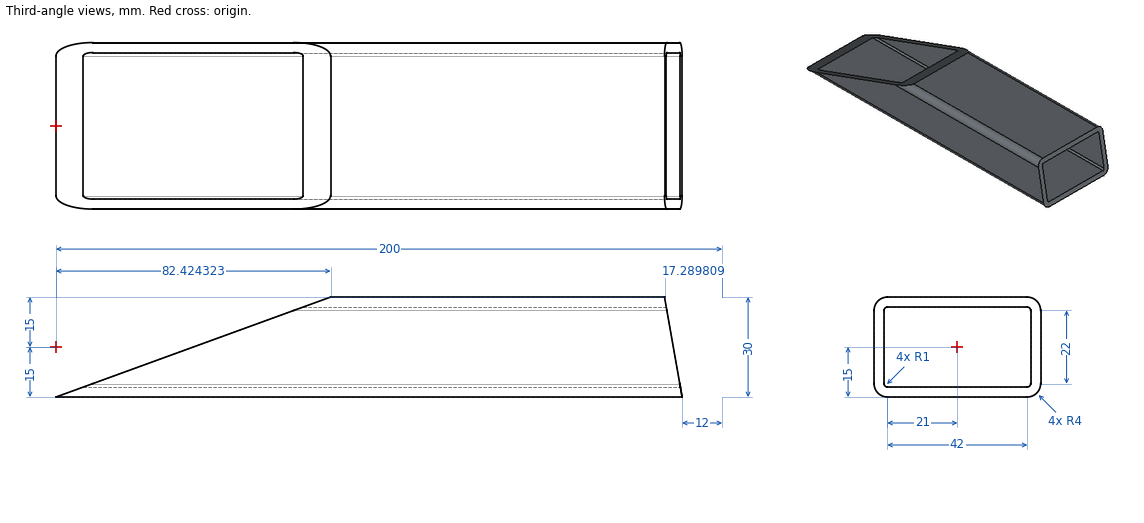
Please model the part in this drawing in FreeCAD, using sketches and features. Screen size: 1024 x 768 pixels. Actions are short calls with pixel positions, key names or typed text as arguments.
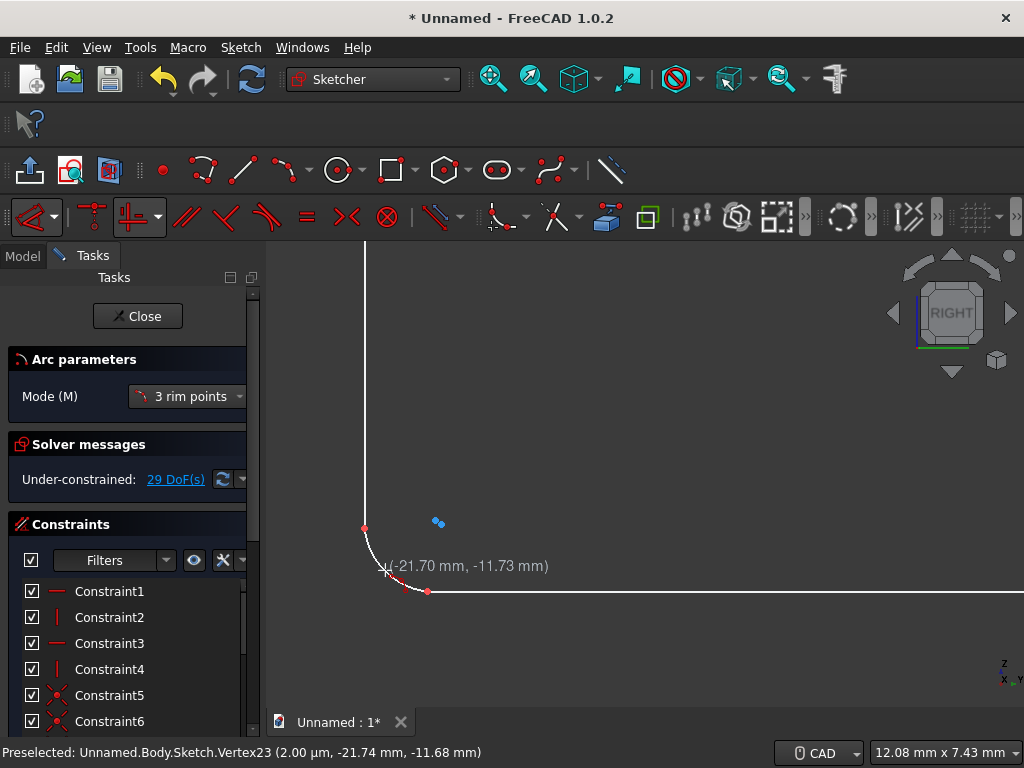
scroll(393, 574, down, 10)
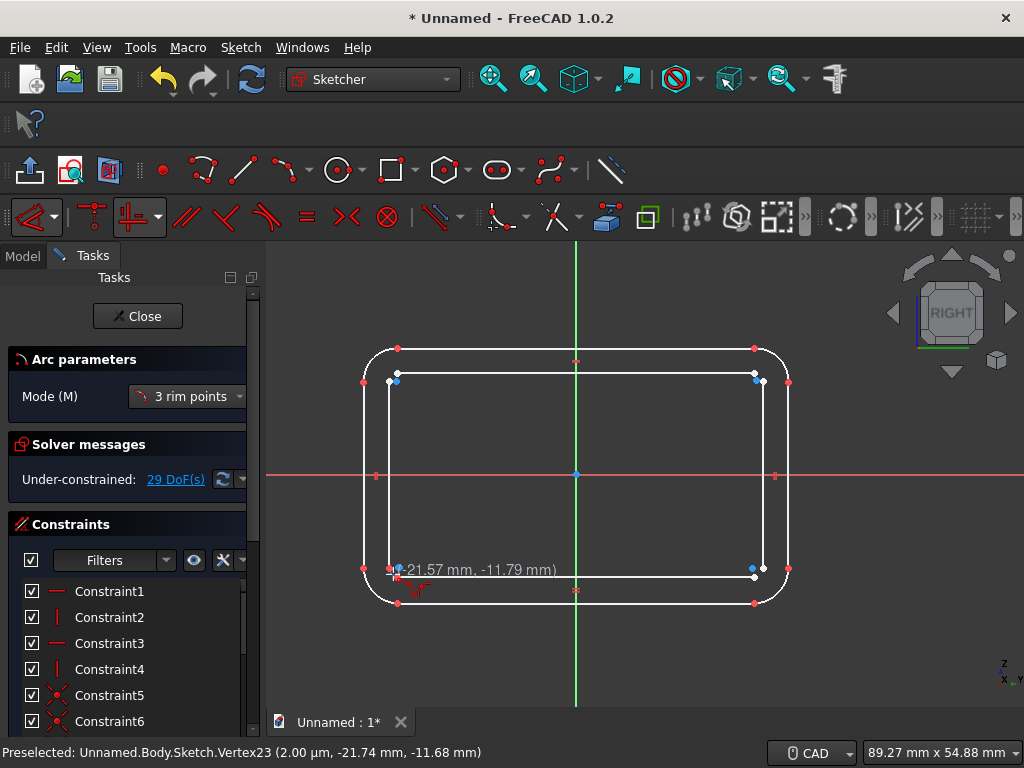
scroll(390, 381, up, 4)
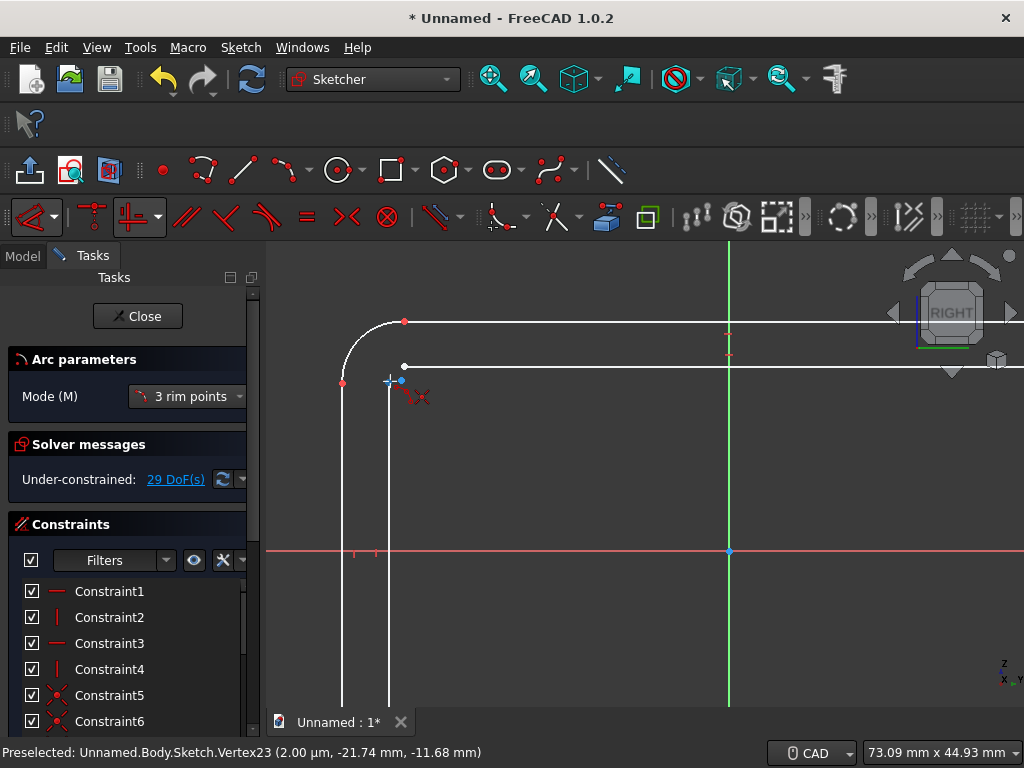
click(388, 382)
click(407, 363)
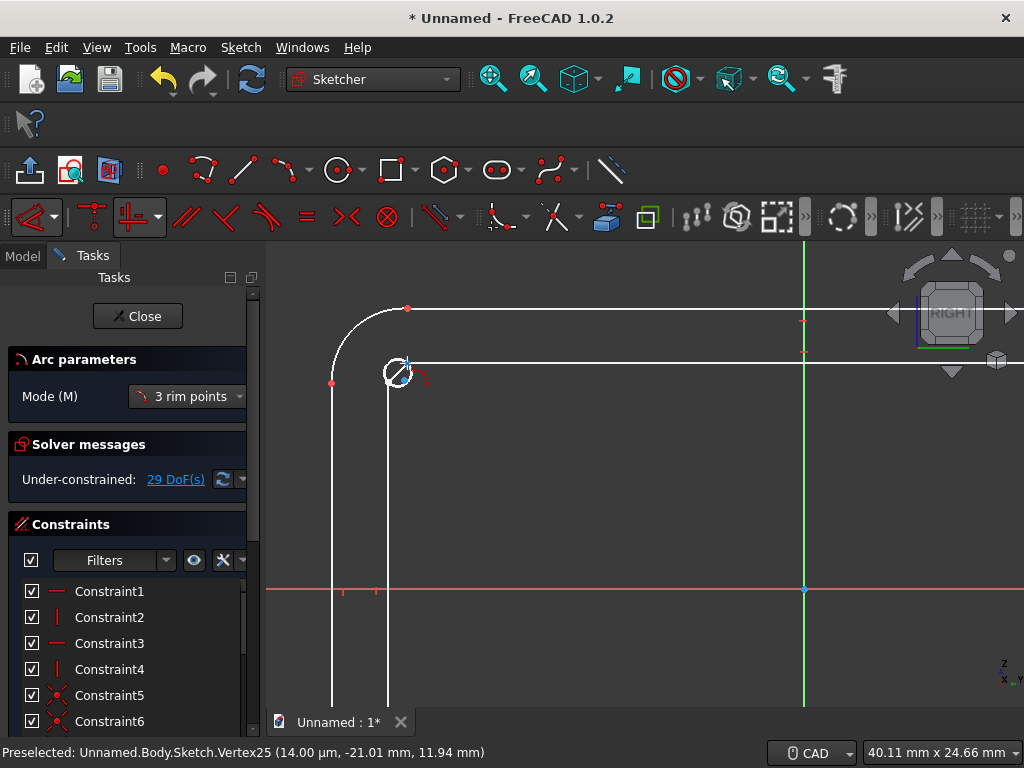
scroll(394, 368, up, 6)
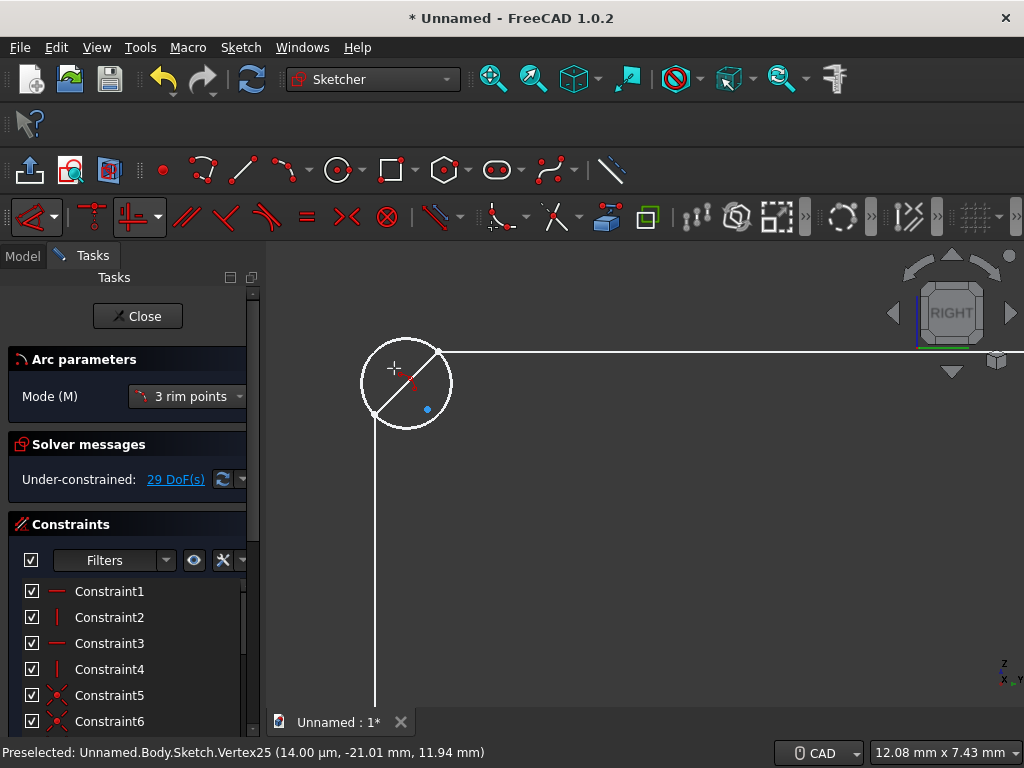
click(394, 367)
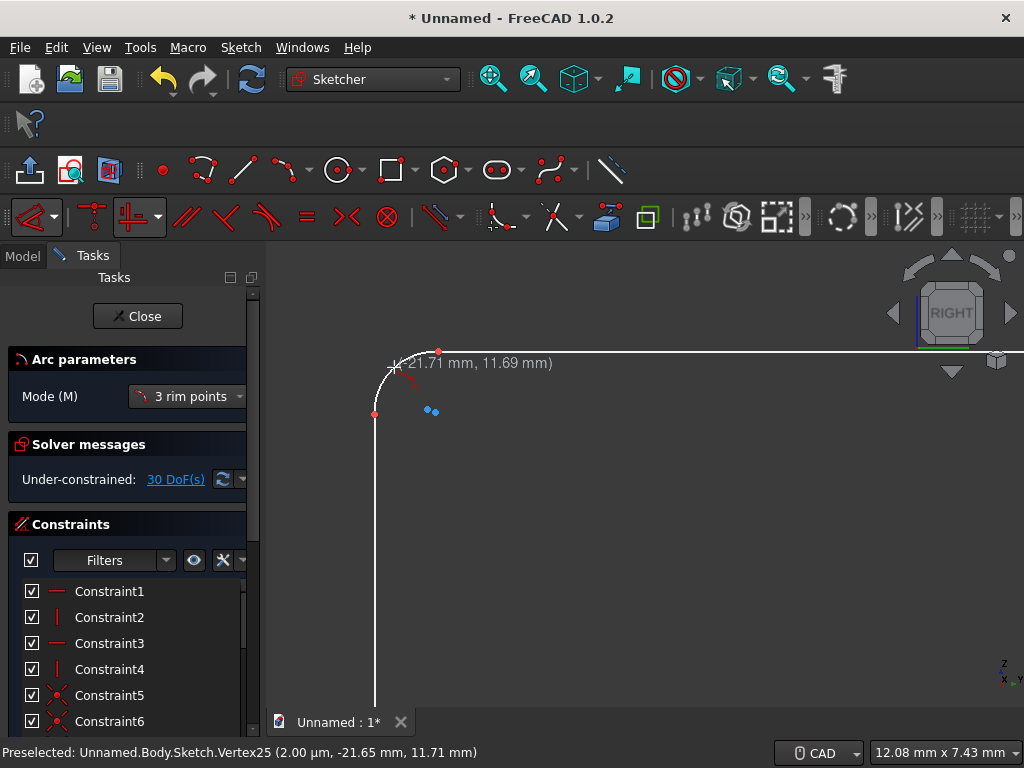
scroll(392, 376, down, 10)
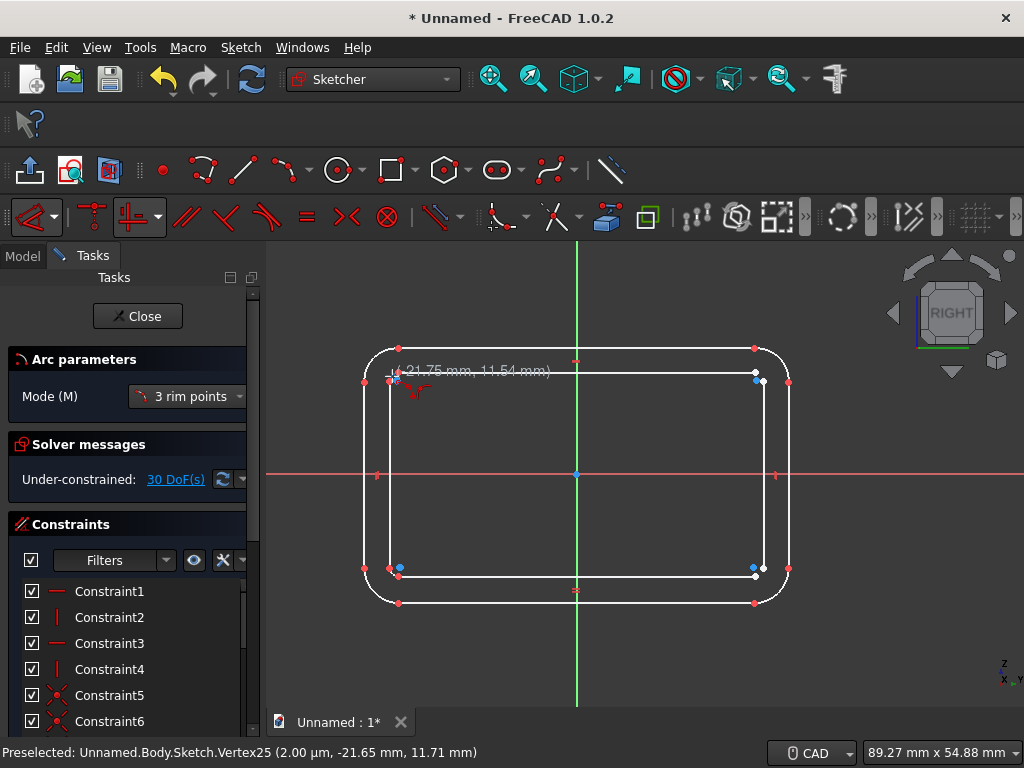
scroll(755, 373, up, 4)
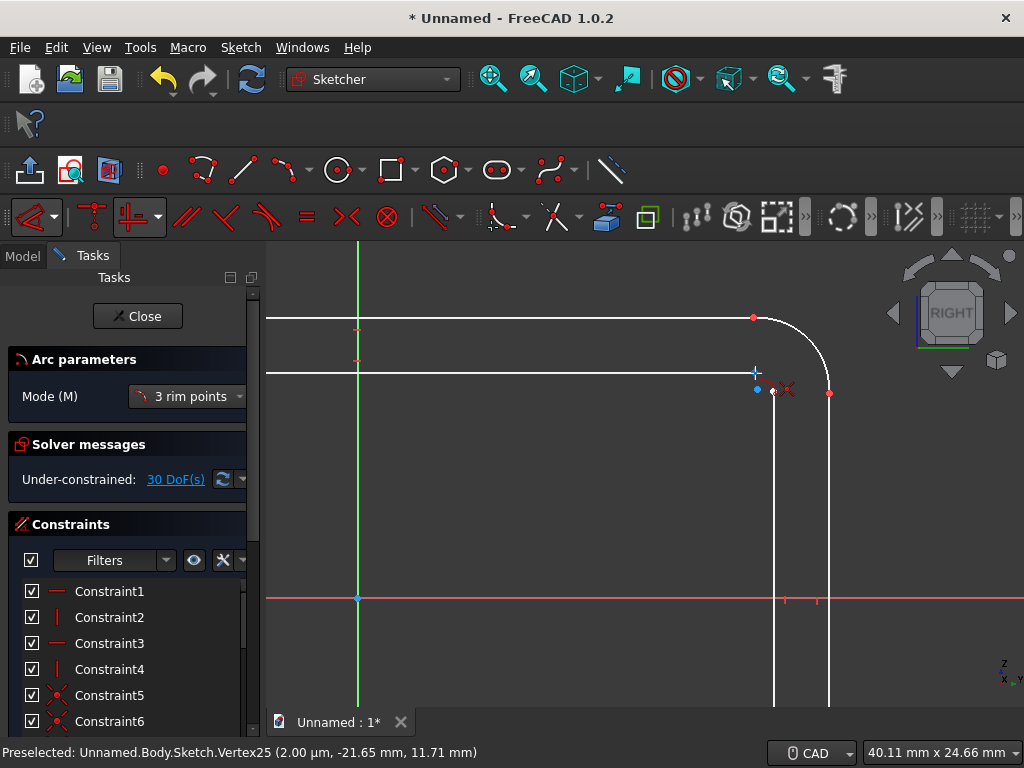
click(755, 373)
click(774, 392)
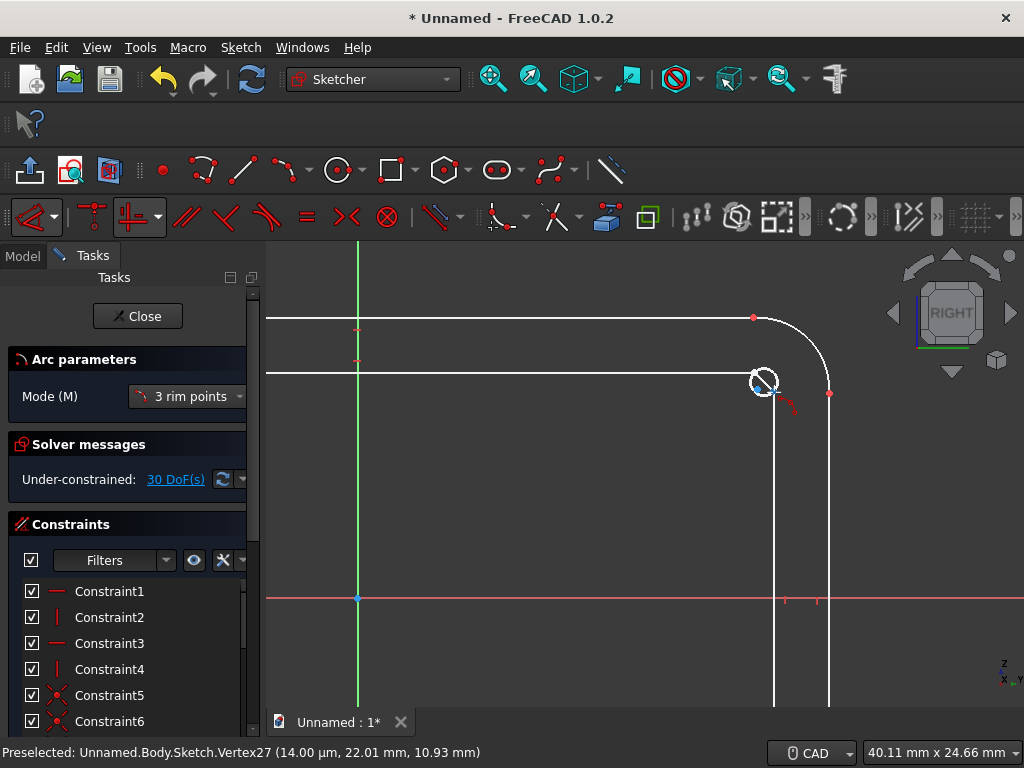
scroll(768, 377, up, 6)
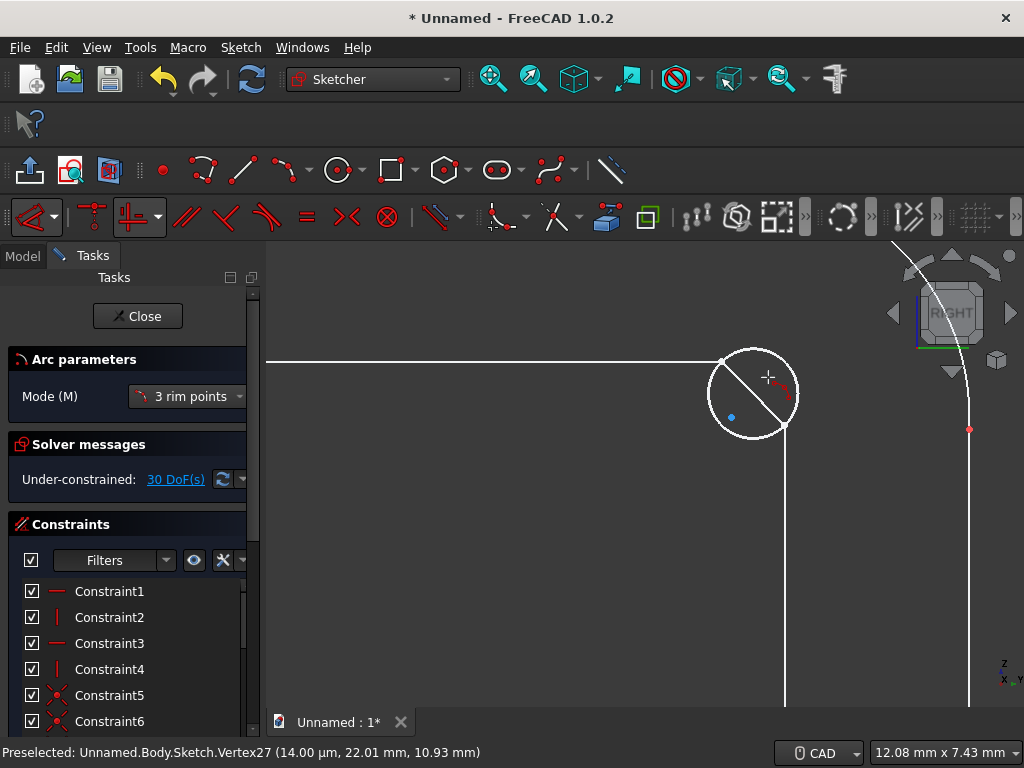
click(766, 377)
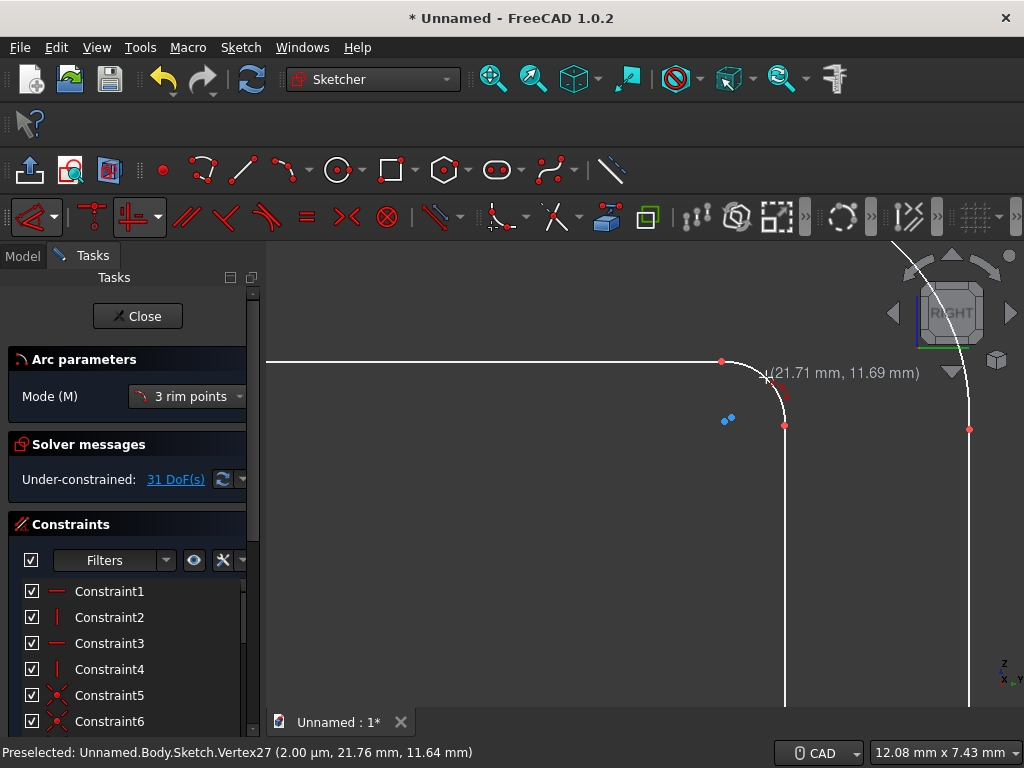
scroll(760, 374, down, 10)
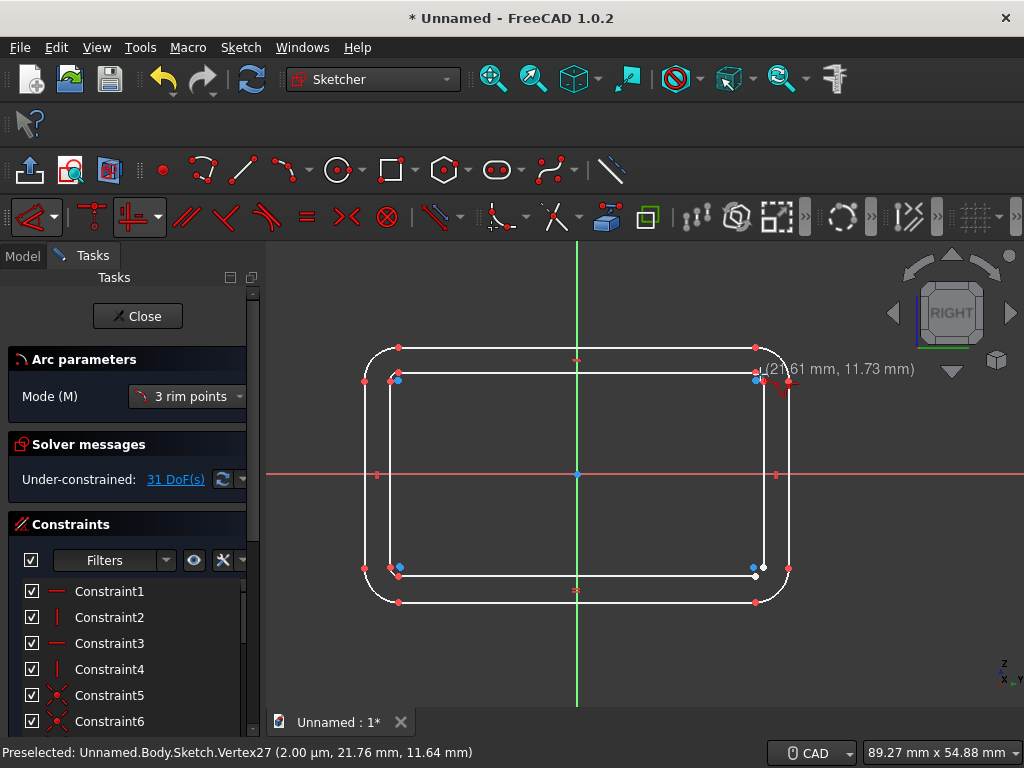
scroll(764, 567, up, 4)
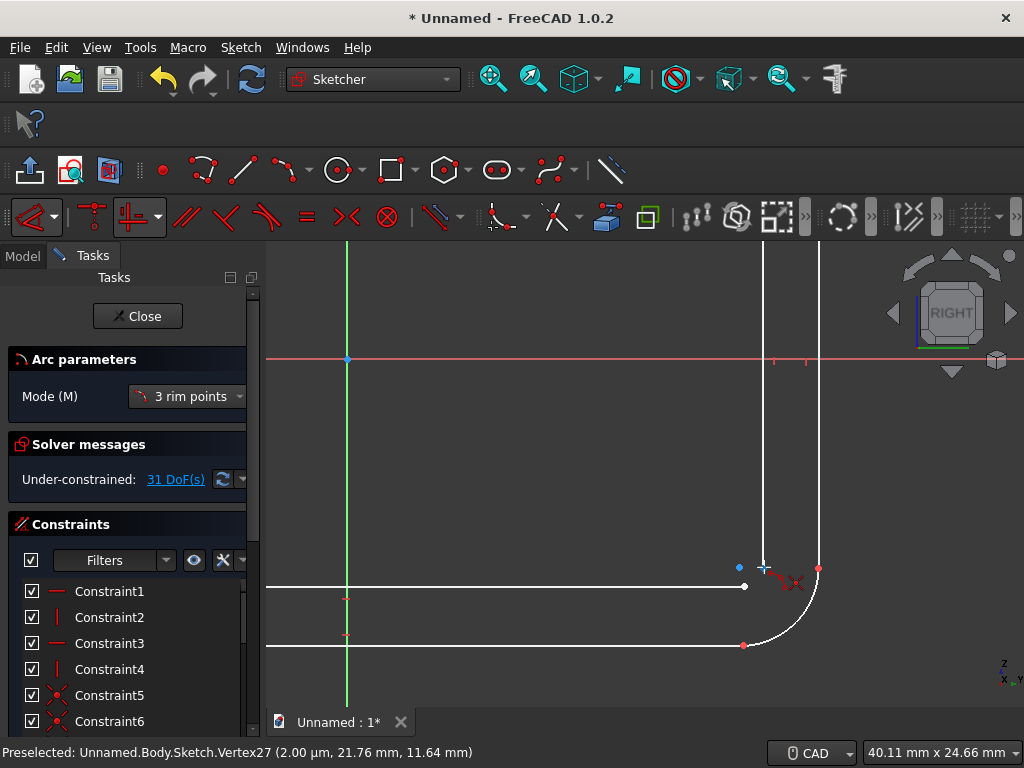
click(763, 568)
click(744, 587)